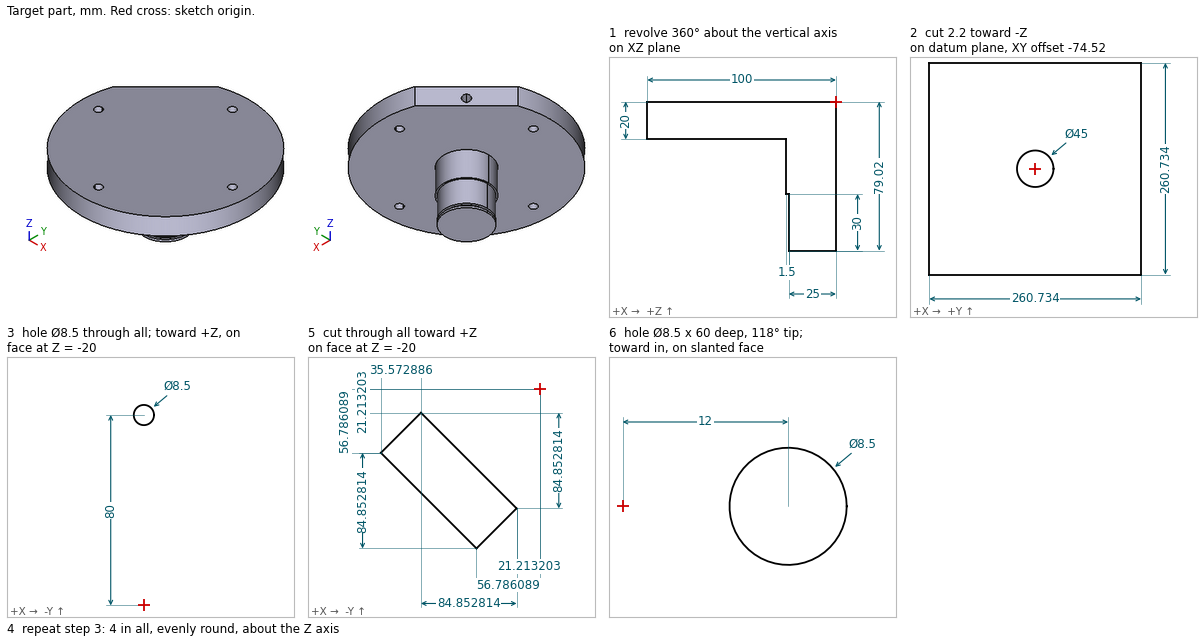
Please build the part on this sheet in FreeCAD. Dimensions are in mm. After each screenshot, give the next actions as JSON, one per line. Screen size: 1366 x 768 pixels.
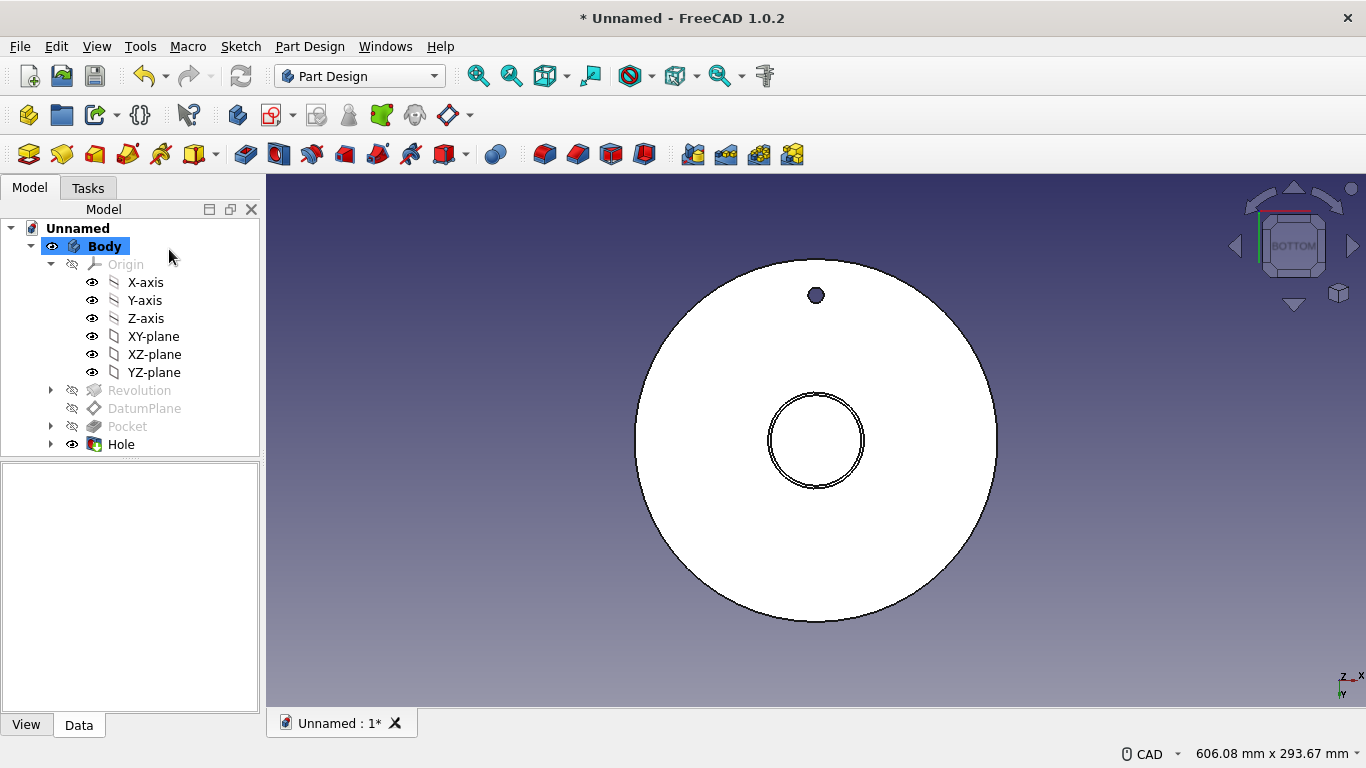
{"action": "left_click", "coordinate": [117, 444]}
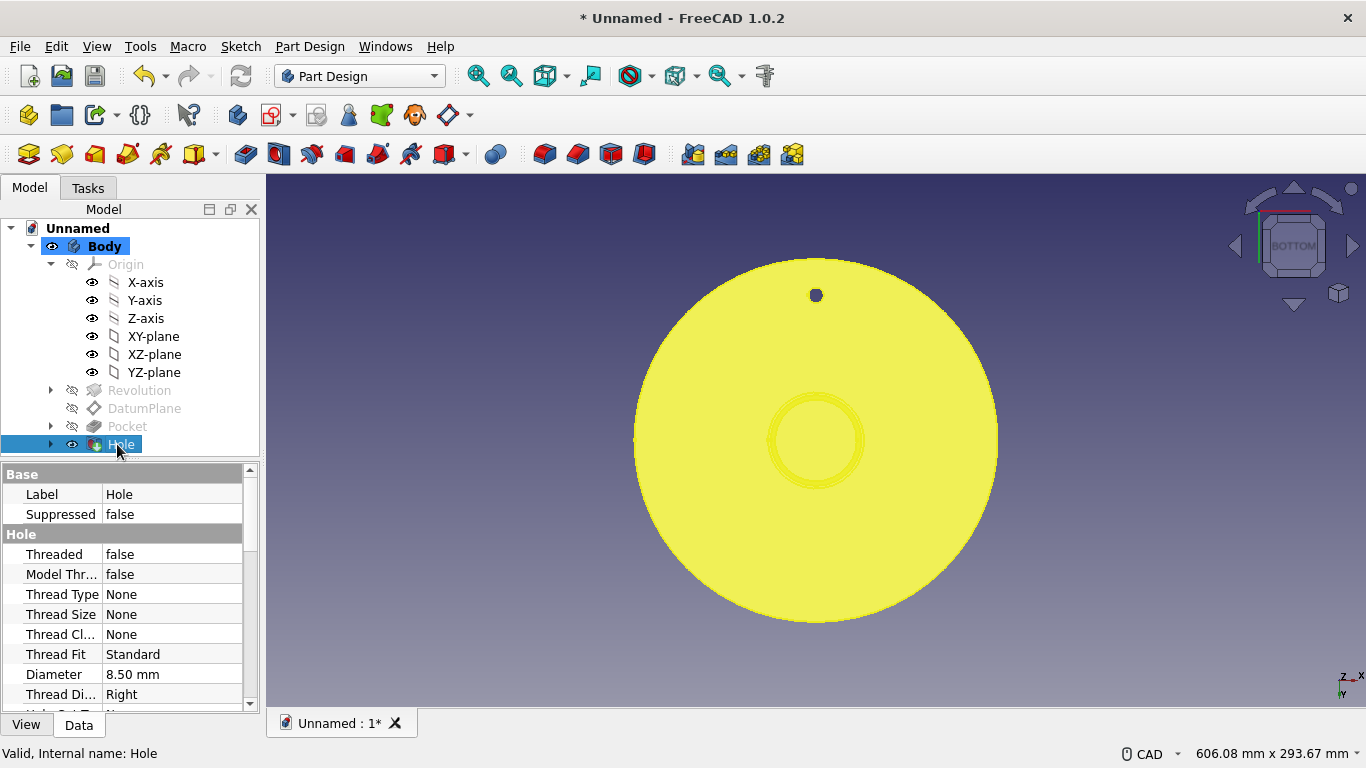
{"action": "left_click", "coordinate": [759, 154]}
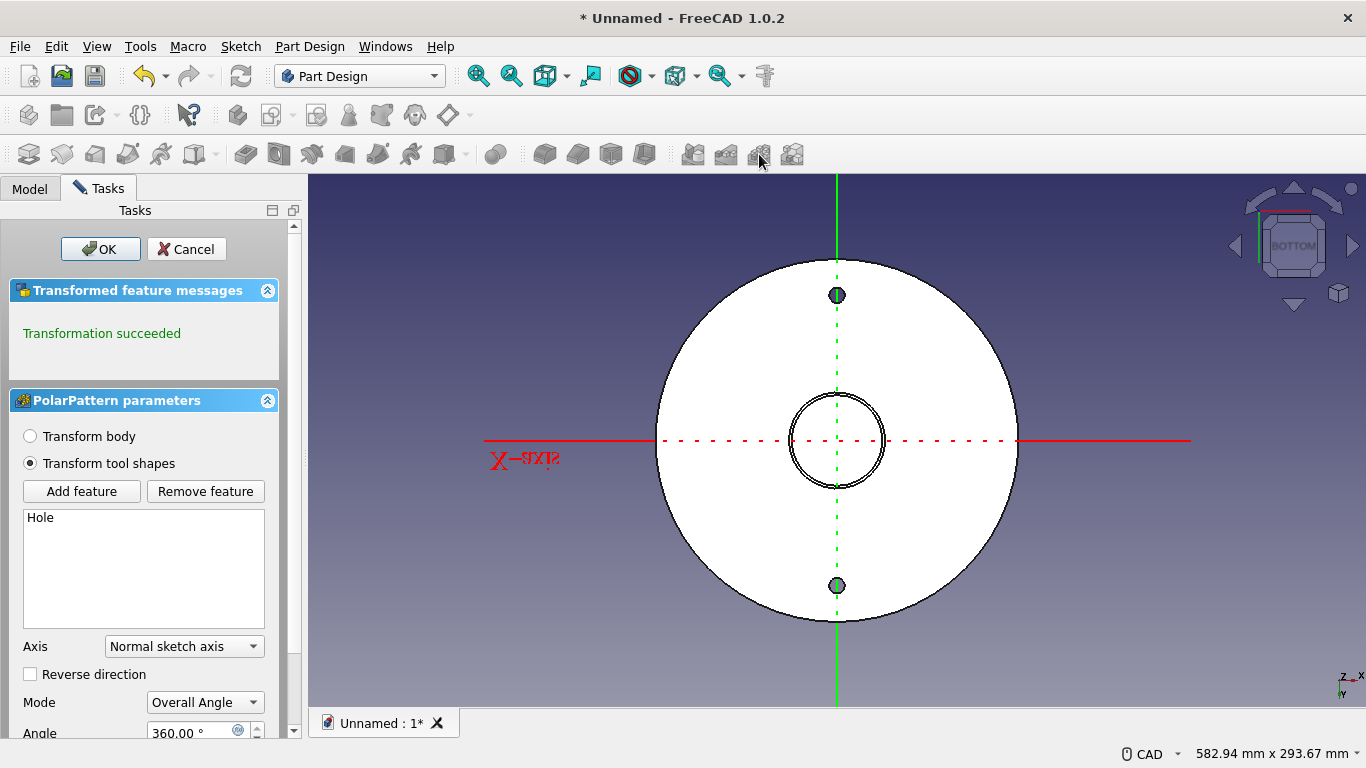
{"action": "left_click", "coordinate": [185, 646]}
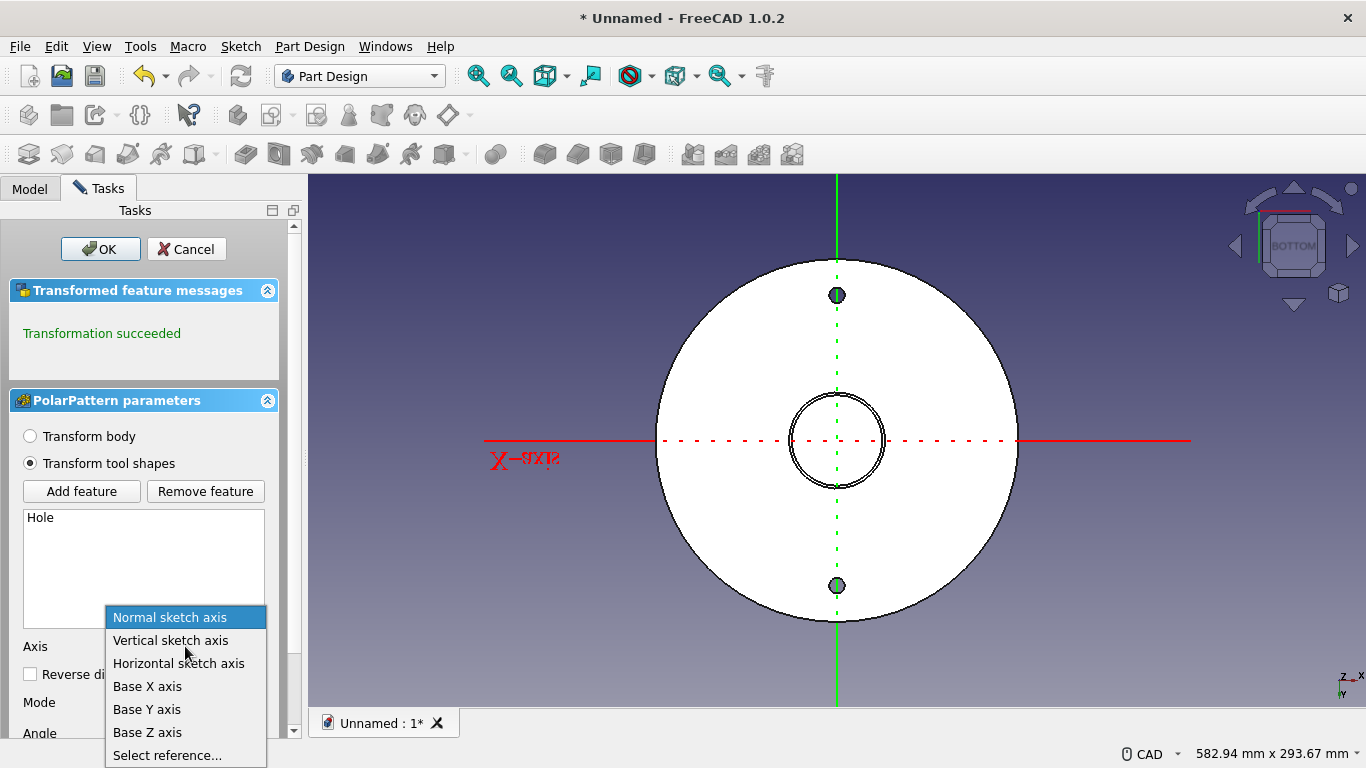
{"action": "left_click", "coordinate": [184, 732]}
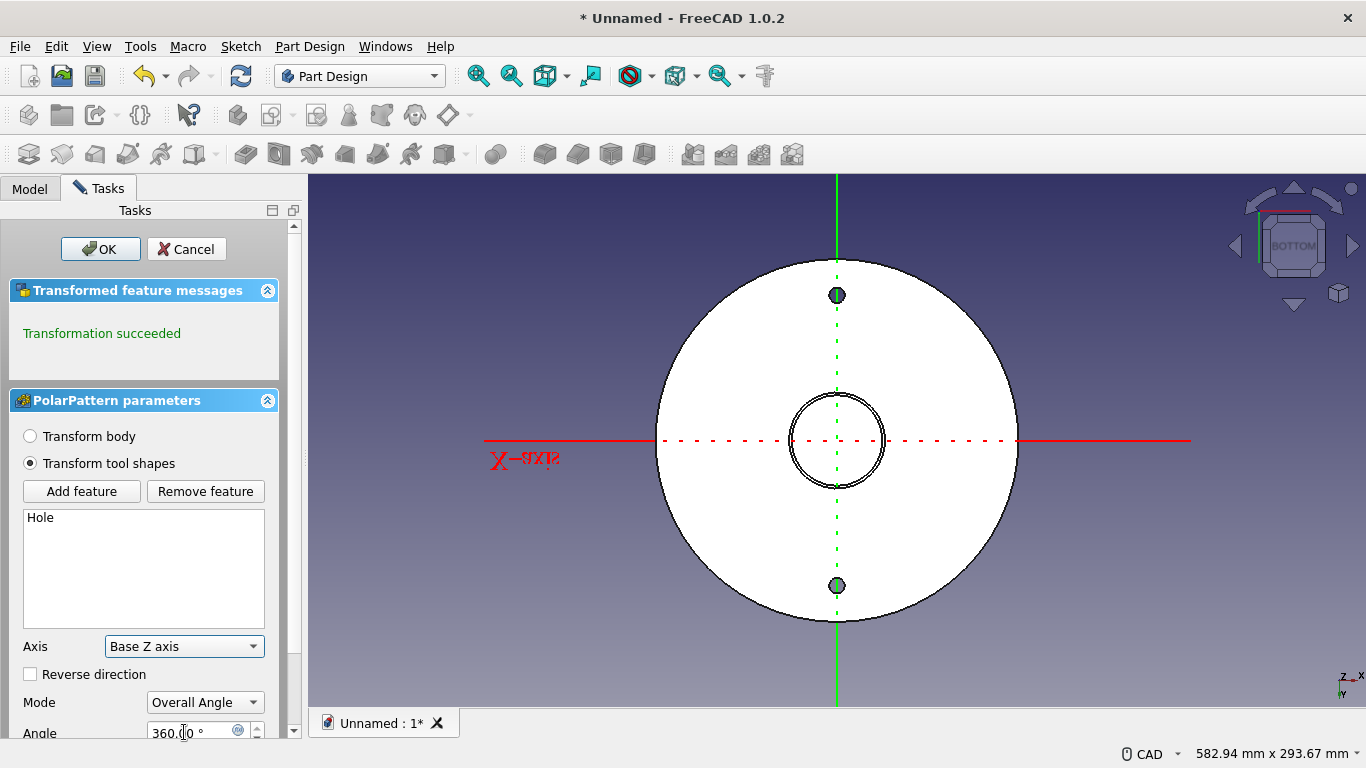
{"action": "scroll", "coordinate": [294, 479], "scroll_direction": "down", "scroll_amount": 2}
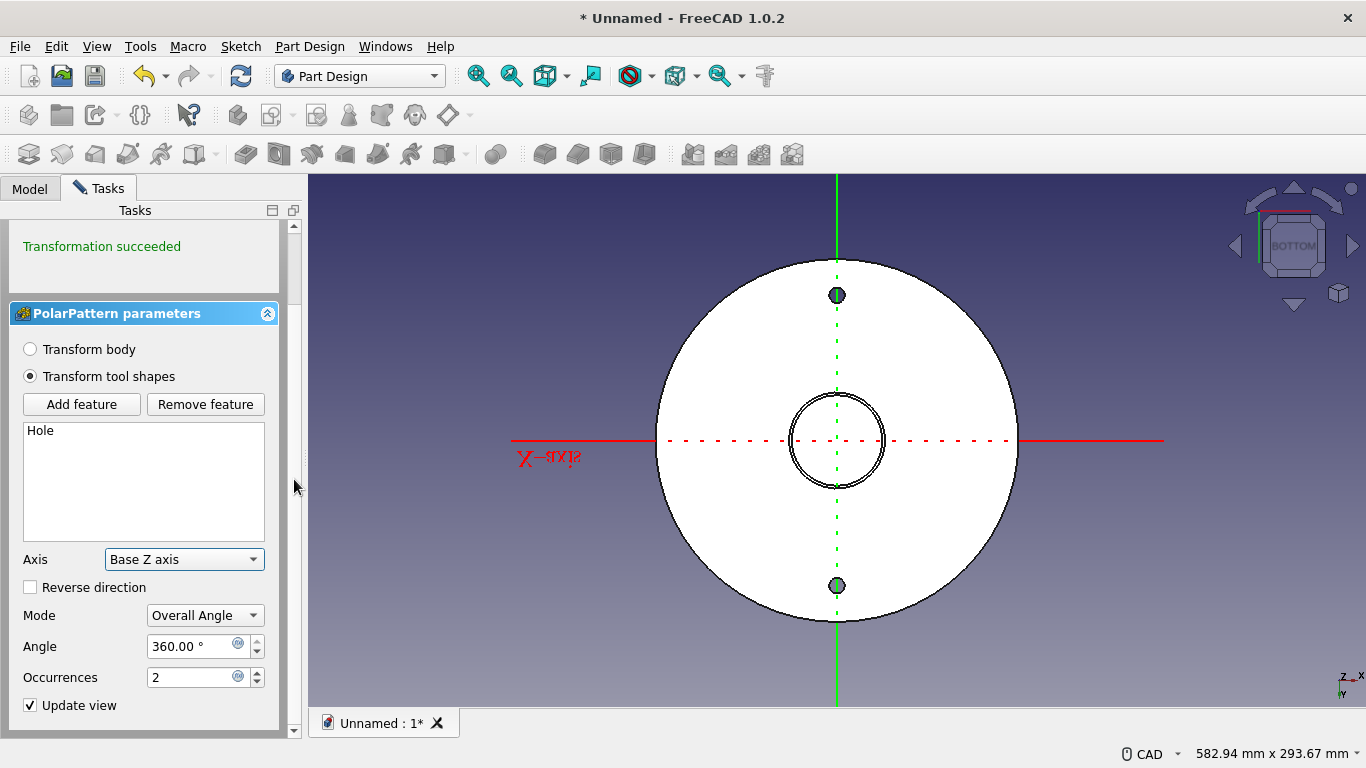
{"action": "triple_click", "coordinate": [199, 678]}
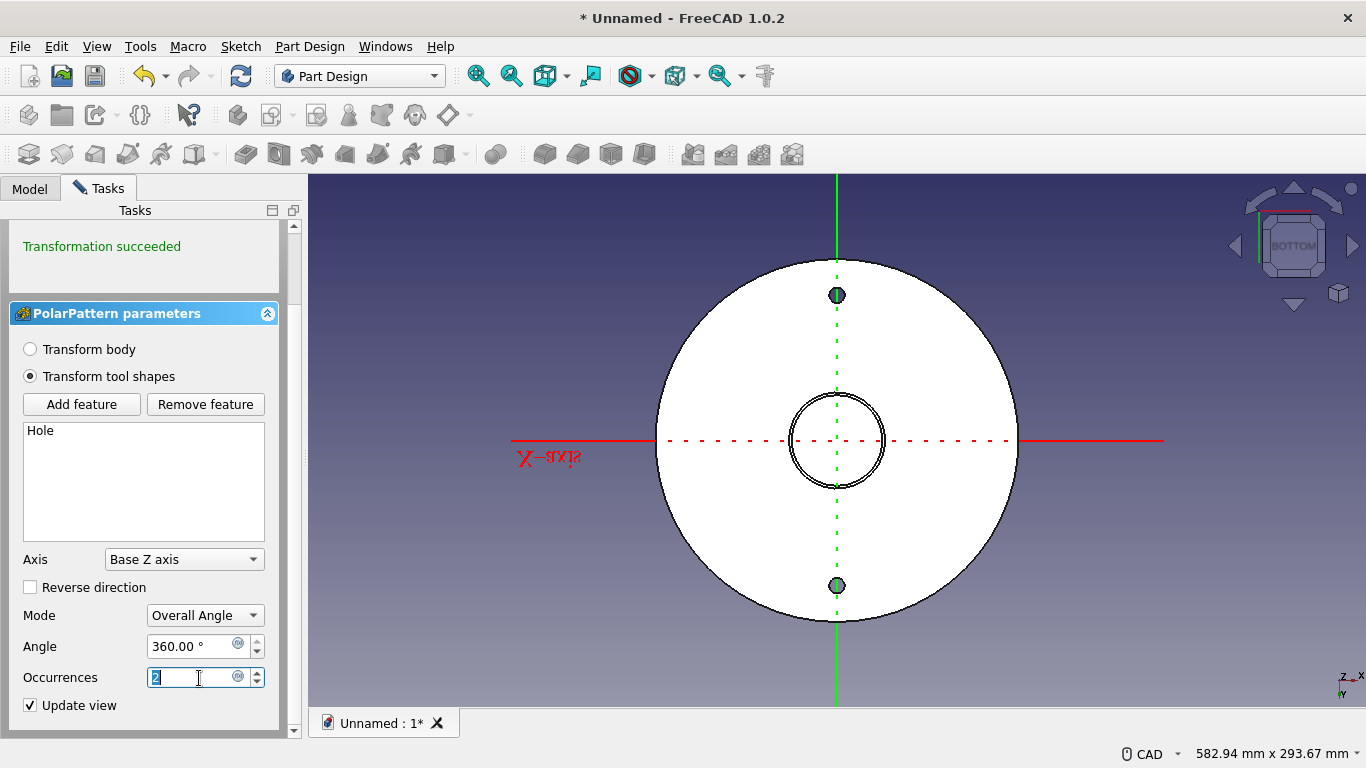
{"action": "type", "text": "4"}
{"action": "key", "text": "Tab"}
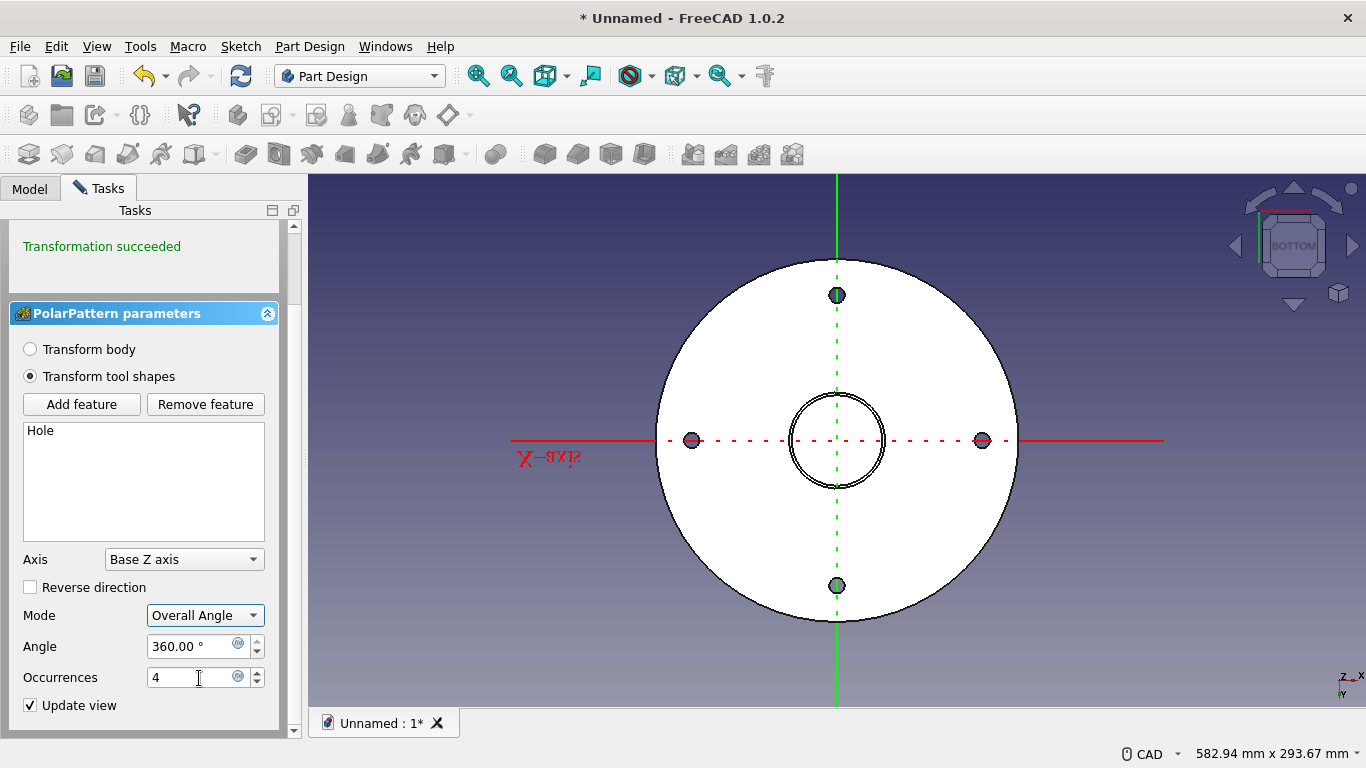
{"action": "scroll", "coordinate": [294, 479], "scroll_direction": "up", "scroll_amount": 3}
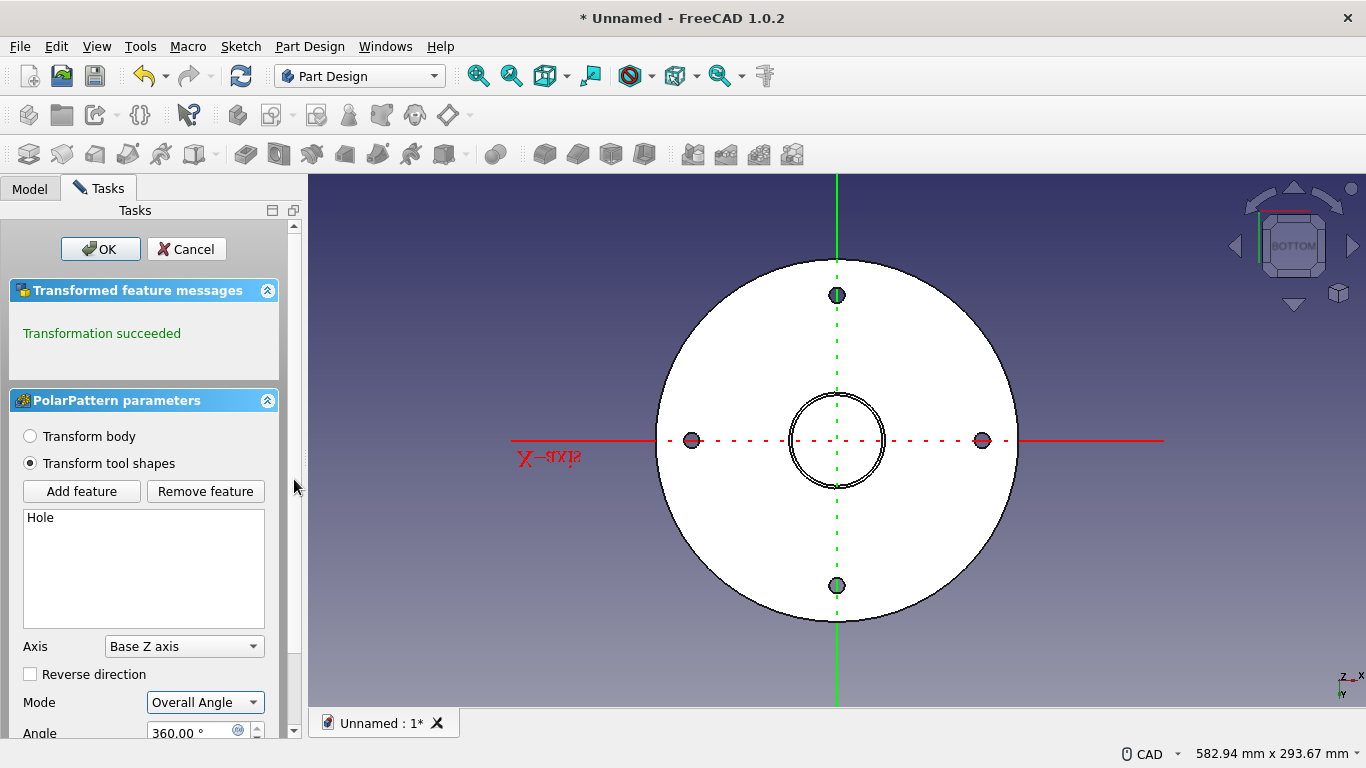
{"action": "left_click", "coordinate": [101, 249]}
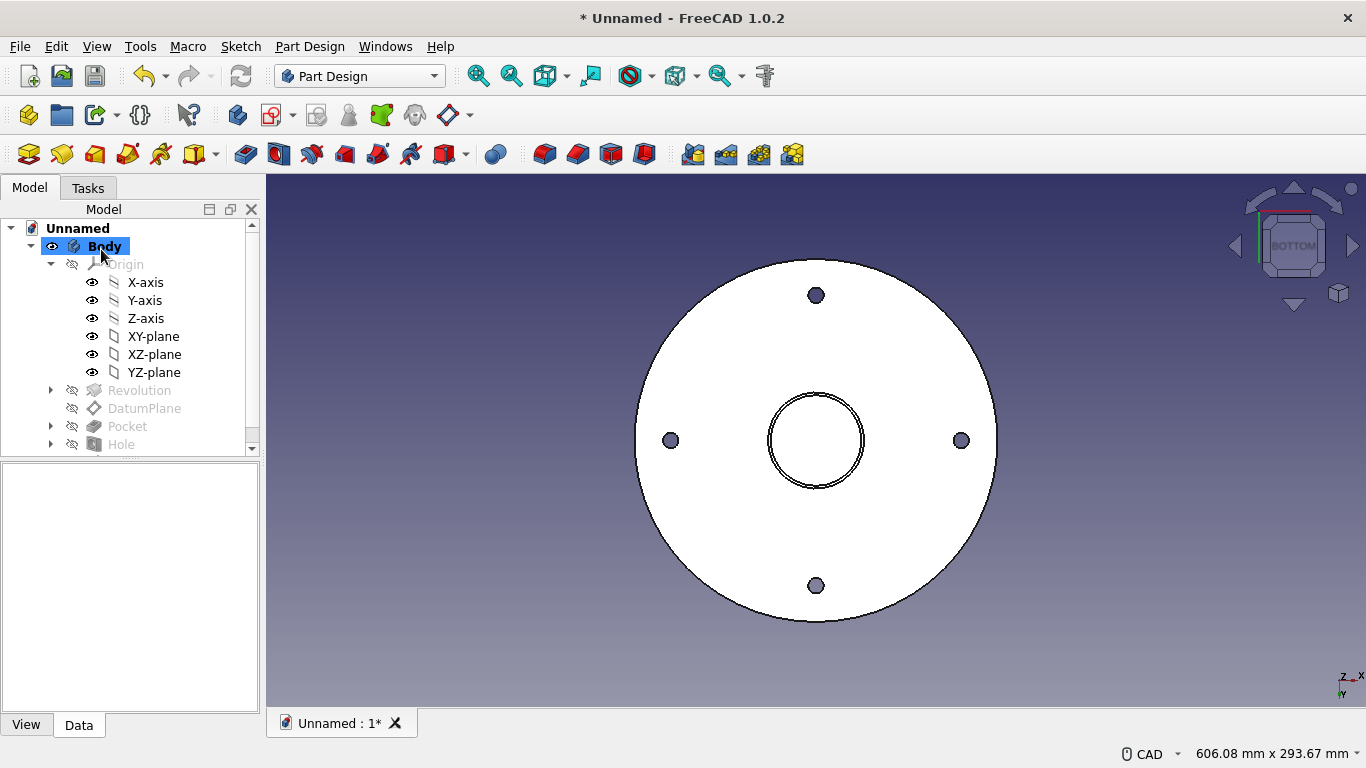
{"action": "left_click", "coordinate": [712, 388]}